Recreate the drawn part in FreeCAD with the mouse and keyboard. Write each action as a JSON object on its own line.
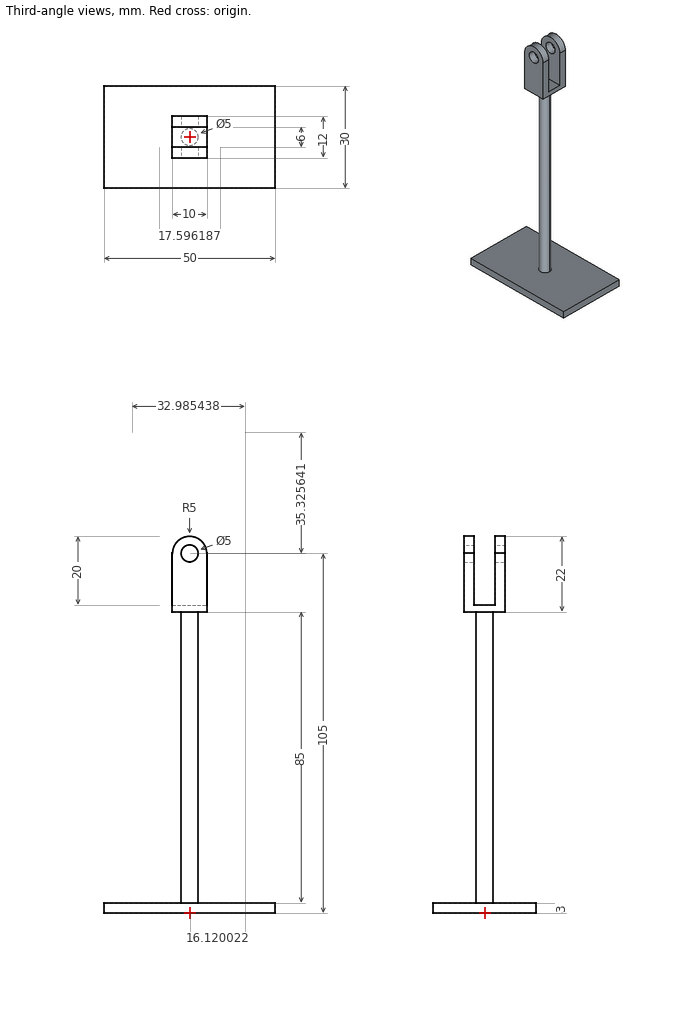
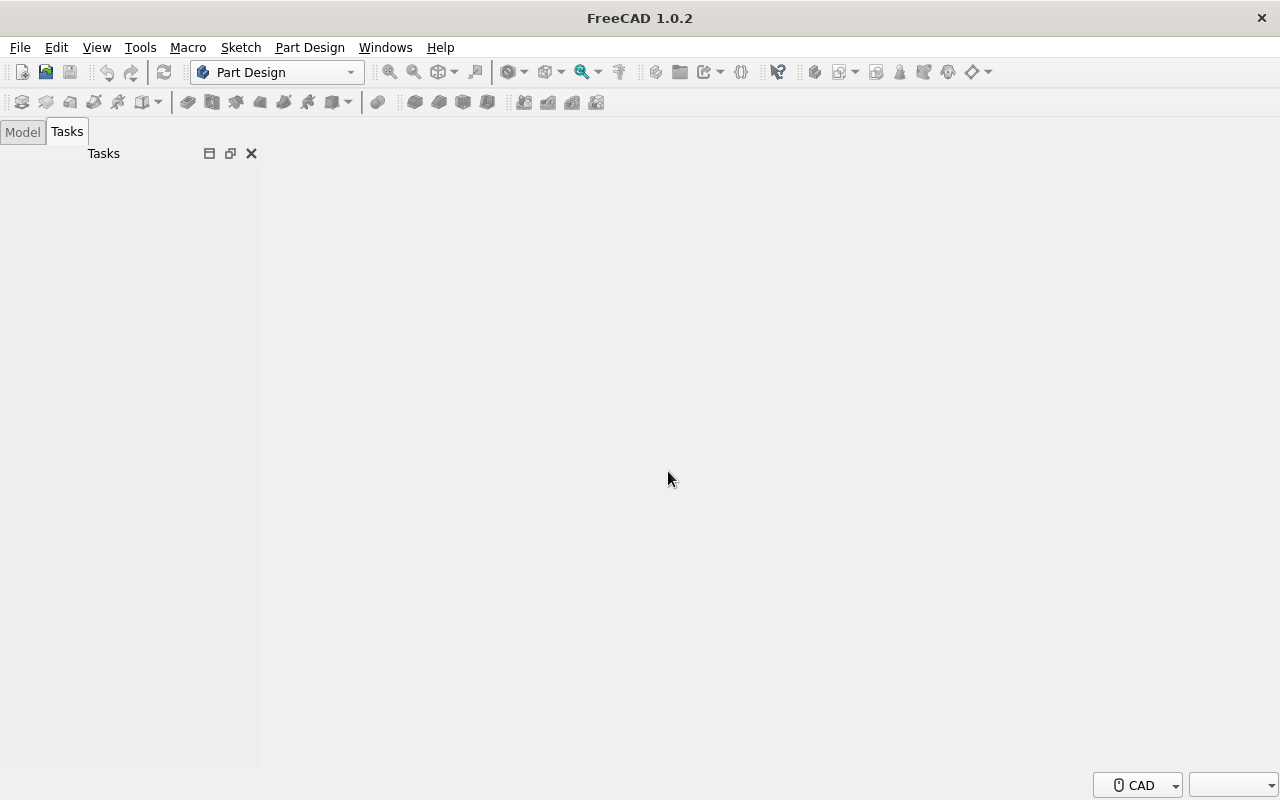
{"action": "left_click", "coordinate": [22, 72]}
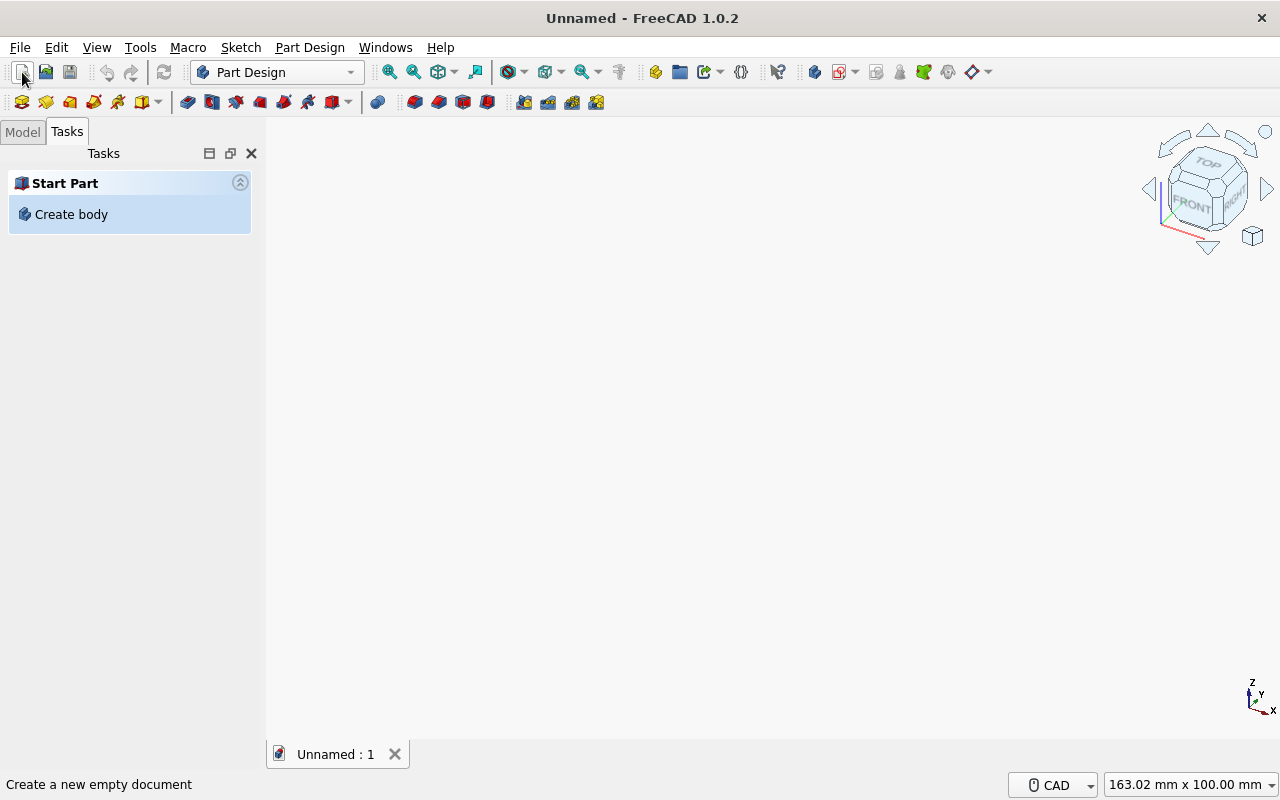
{"action": "left_click", "coordinate": [840, 72]}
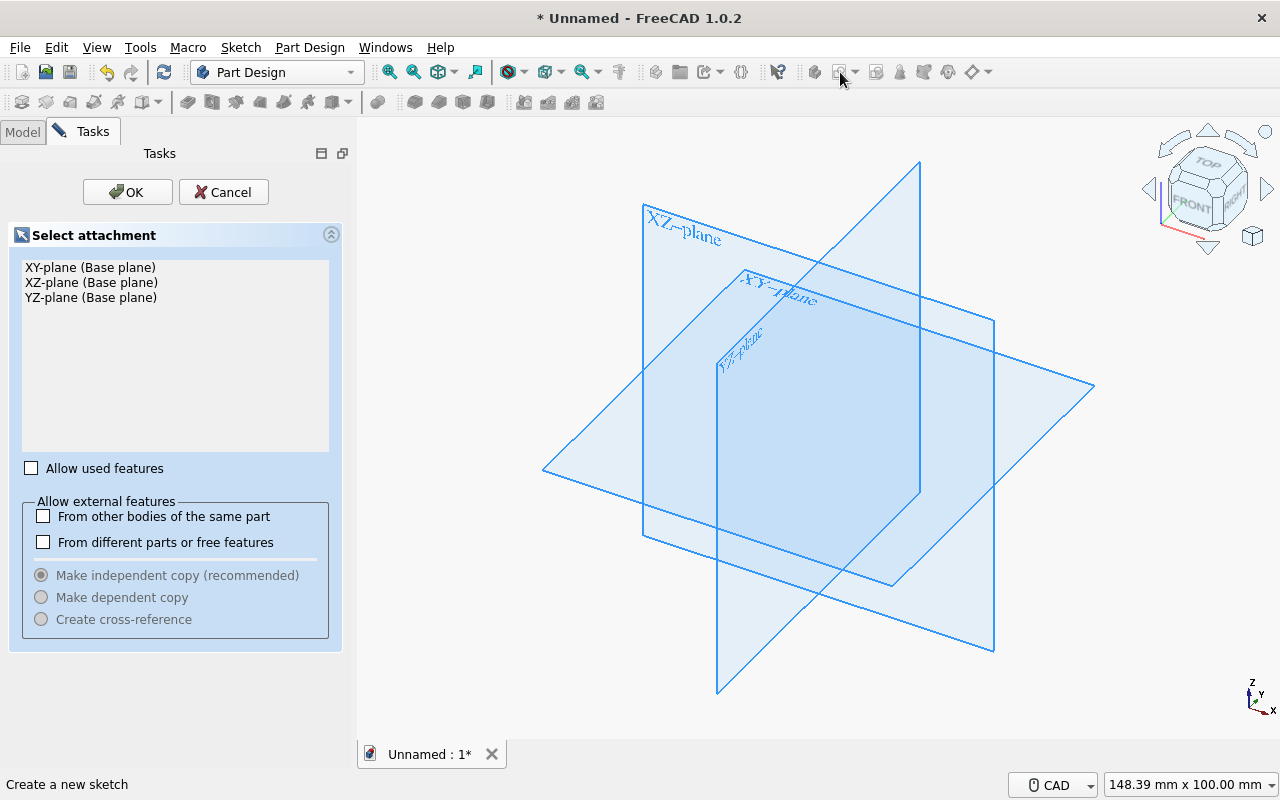
{"action": "left_click", "coordinate": [82, 268]}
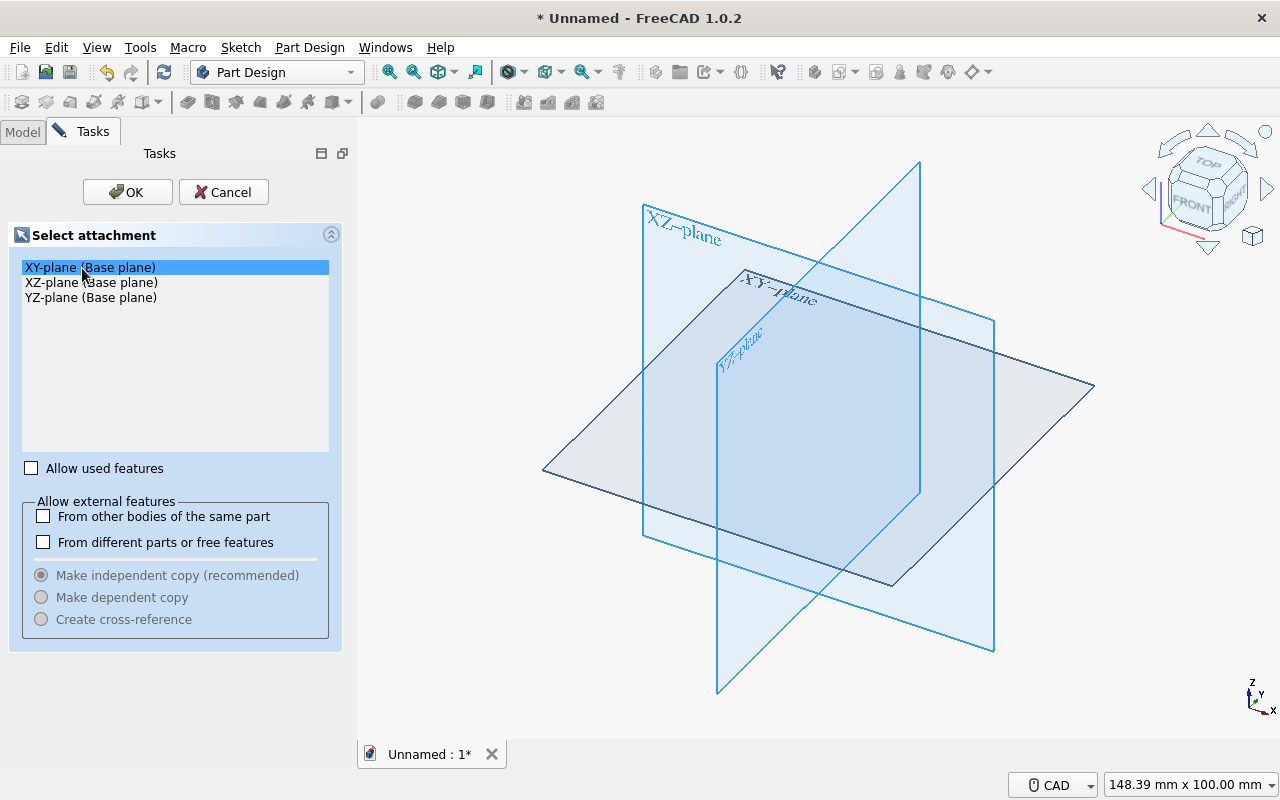
{"action": "left_click", "coordinate": [128, 192]}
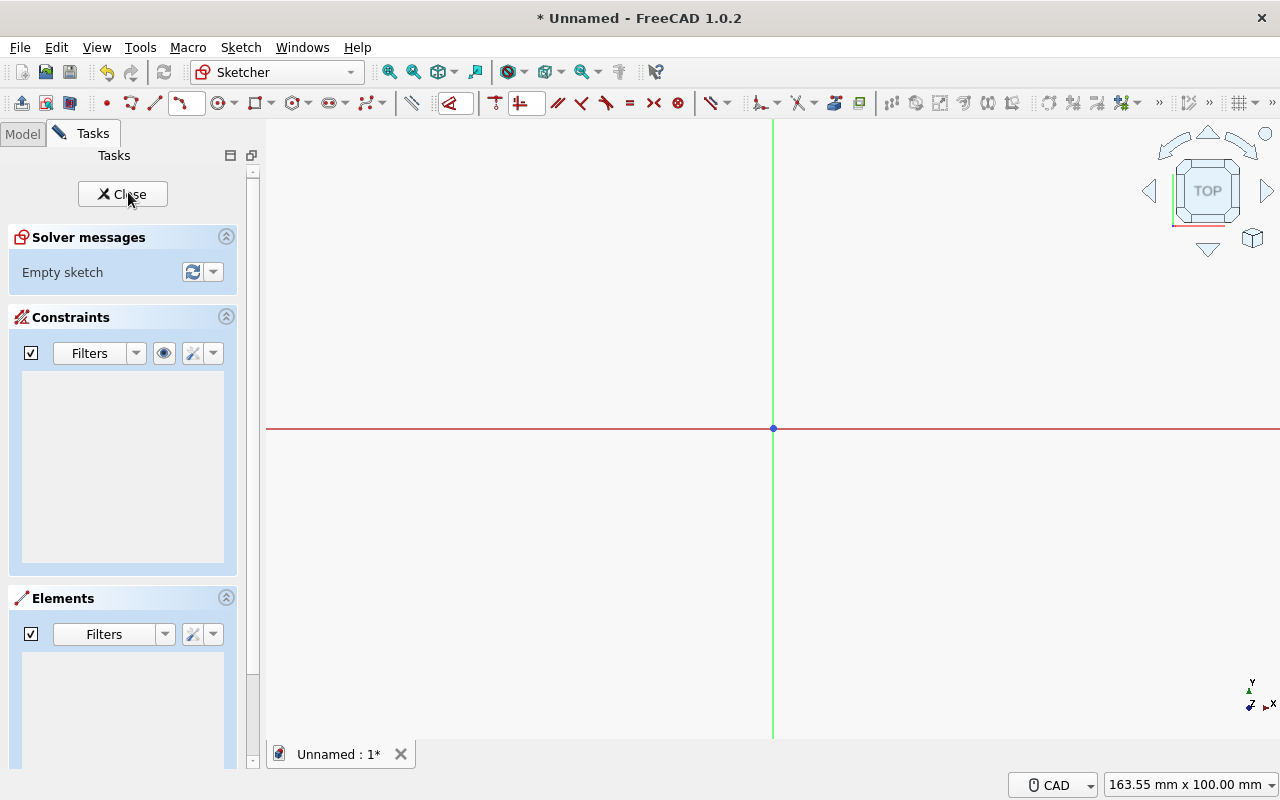
{"action": "scroll", "coordinate": [856, 429], "scroll_direction": "up", "scroll_amount": 3}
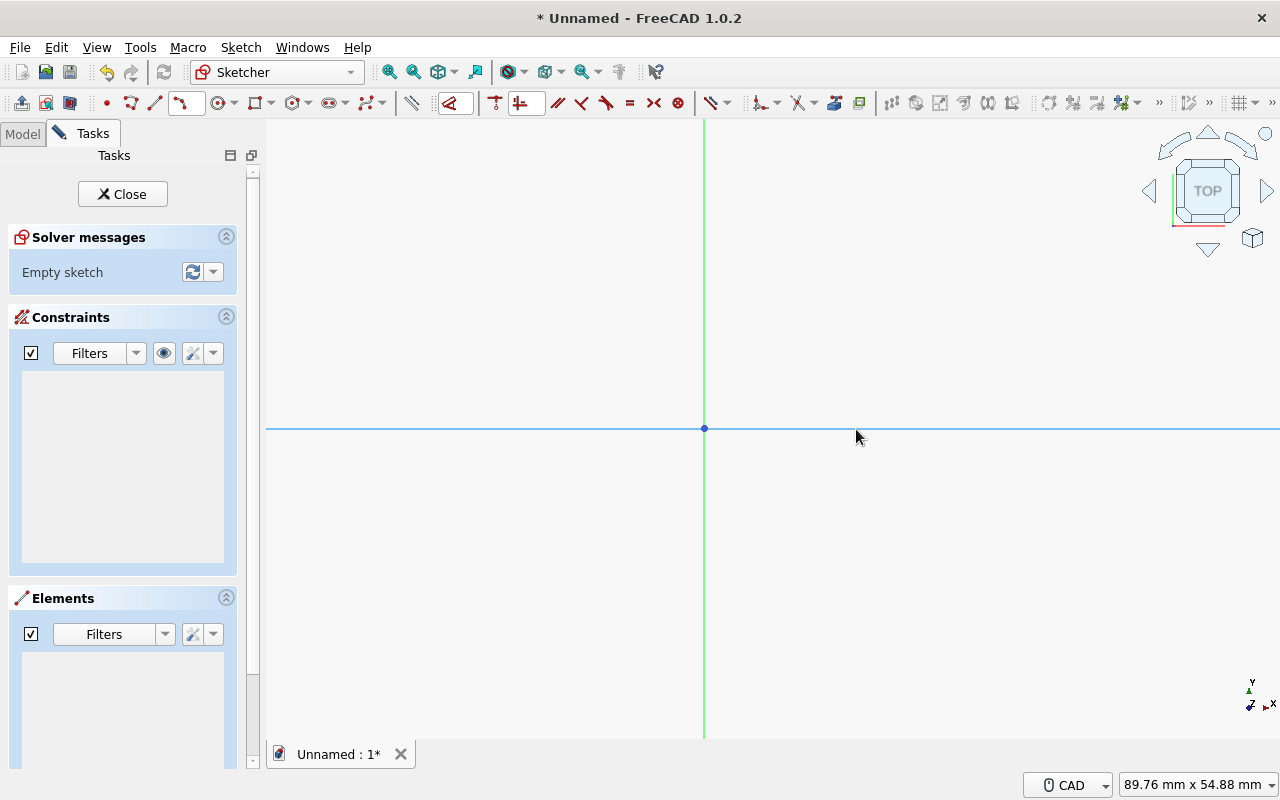
{"action": "left_click", "coordinate": [274, 104]}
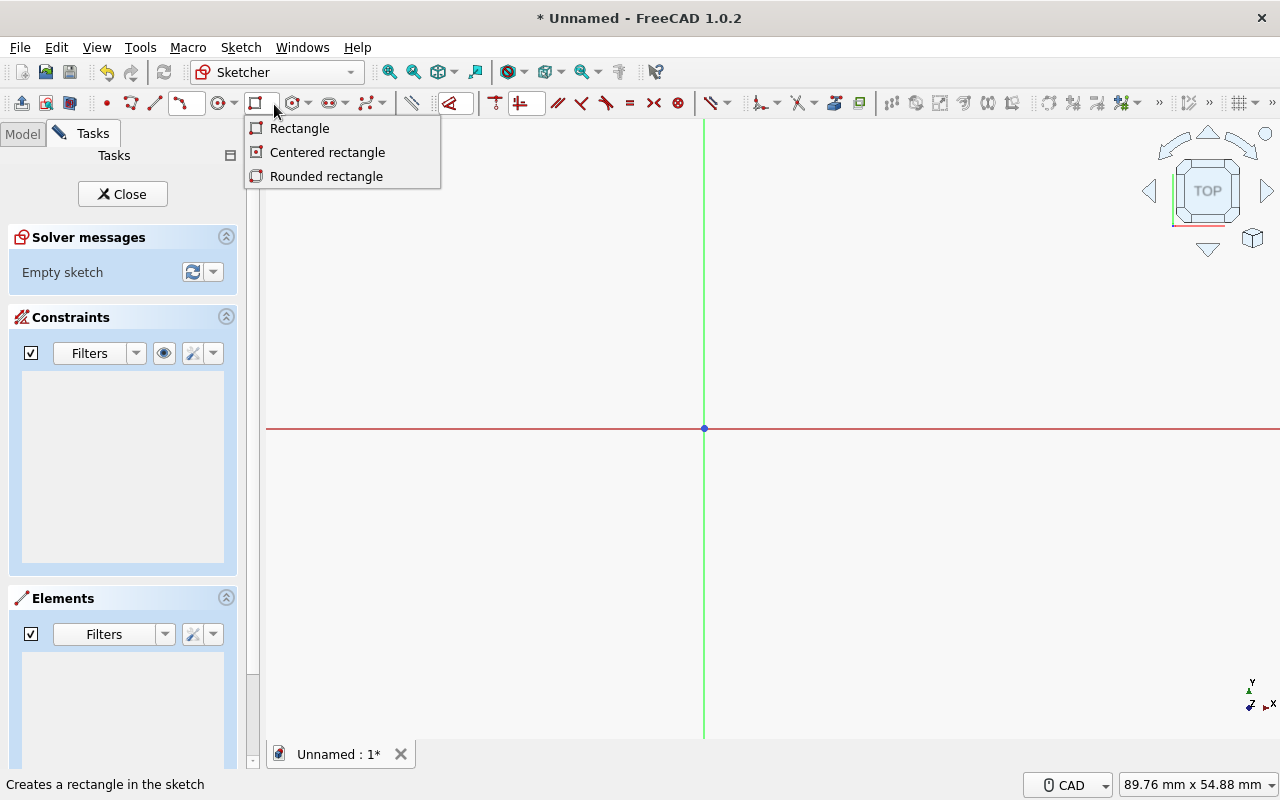
{"action": "left_click", "coordinate": [342, 152]}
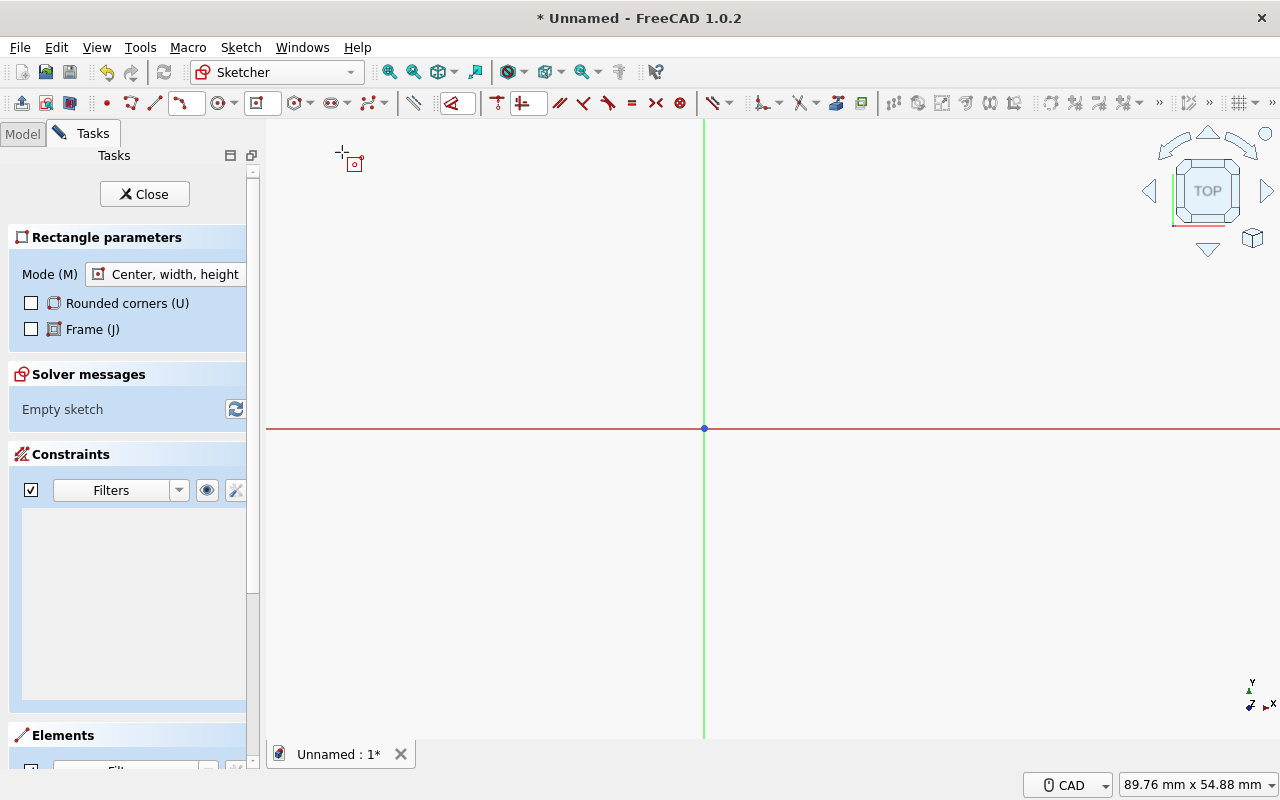
{"action": "left_click", "coordinate": [704, 429]}
{"action": "mouse_move", "coordinate": [987, 259]}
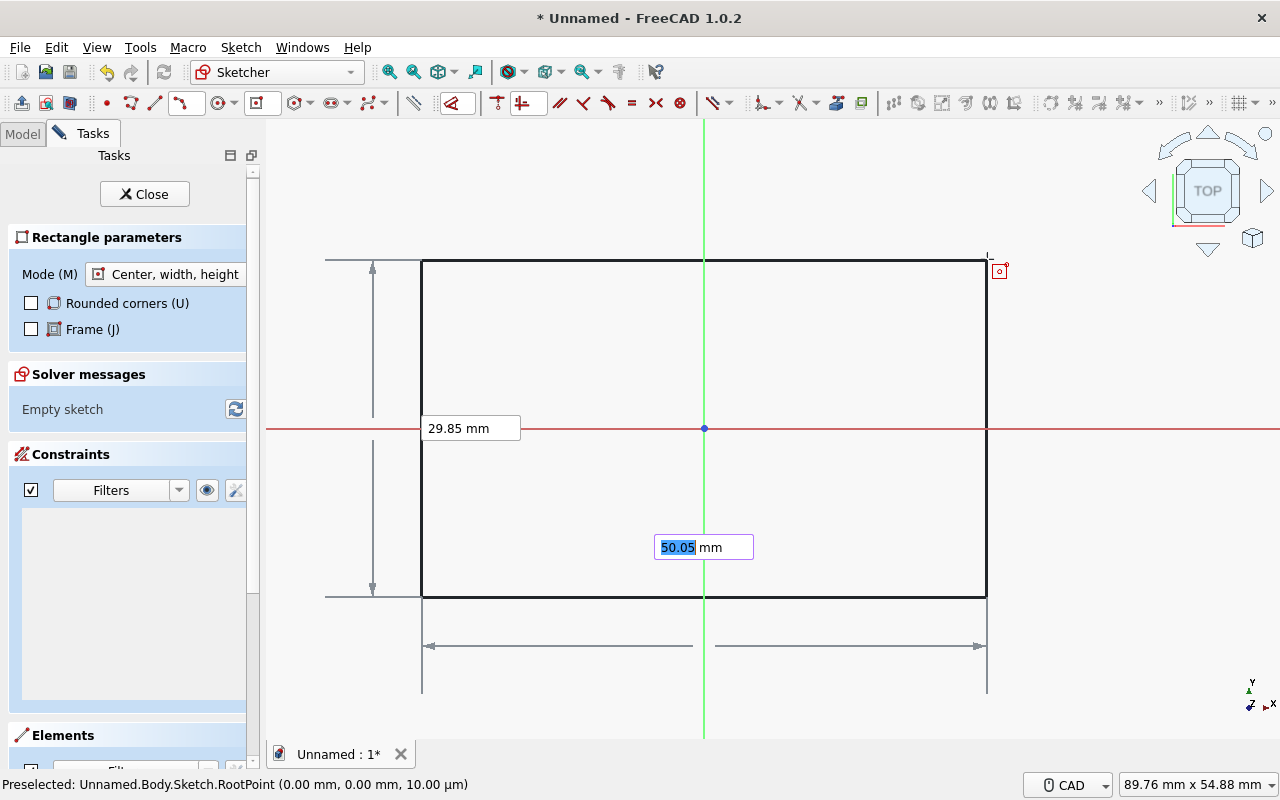
{"action": "type", "text": "50"}
{"action": "key", "text": "Tab"}
{"action": "type", "text": "30"}
{"action": "key", "text": "Return"}
{"action": "key", "text": "Escape"}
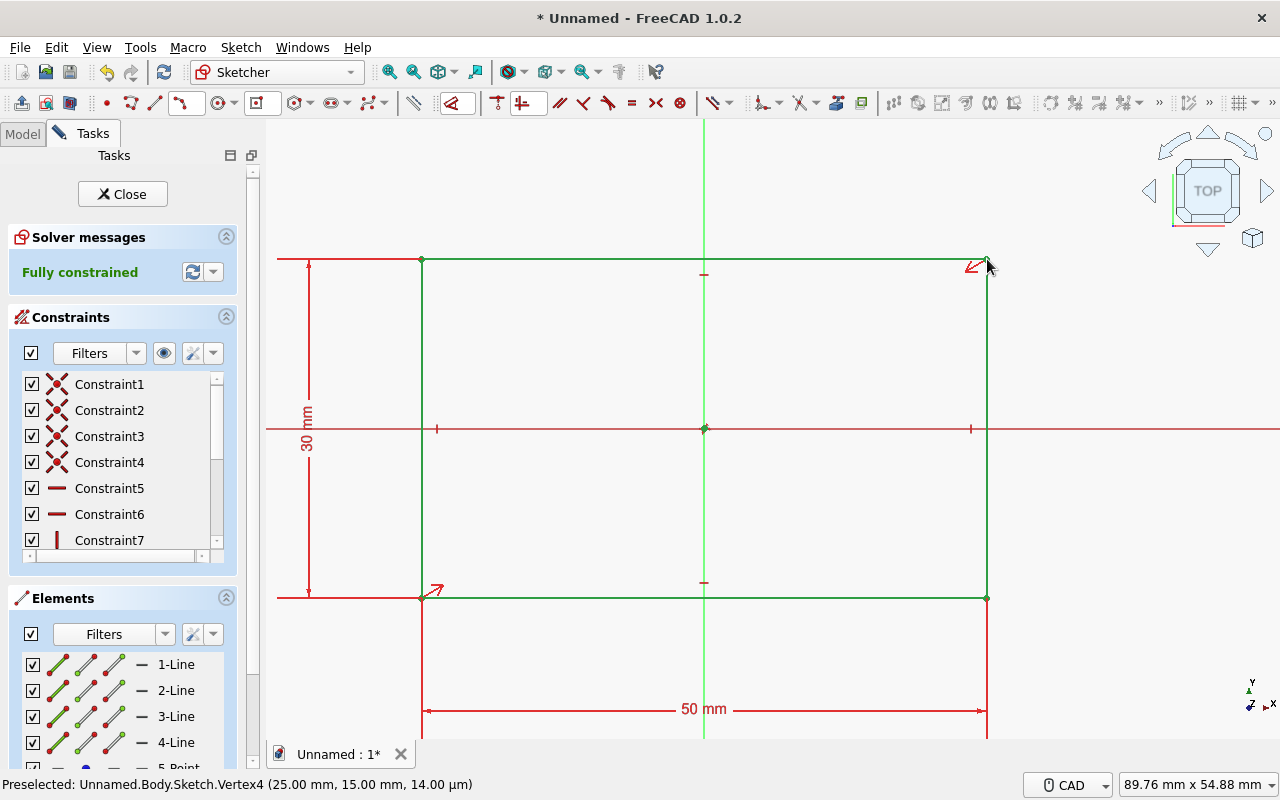
{"action": "left_click", "coordinate": [123, 194]}